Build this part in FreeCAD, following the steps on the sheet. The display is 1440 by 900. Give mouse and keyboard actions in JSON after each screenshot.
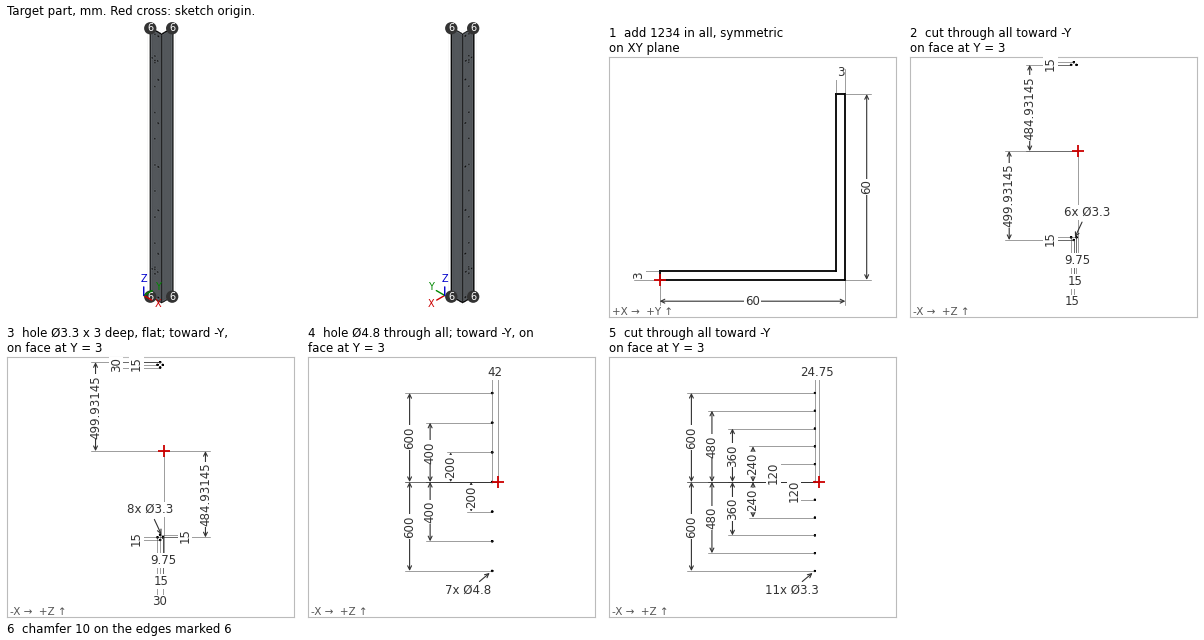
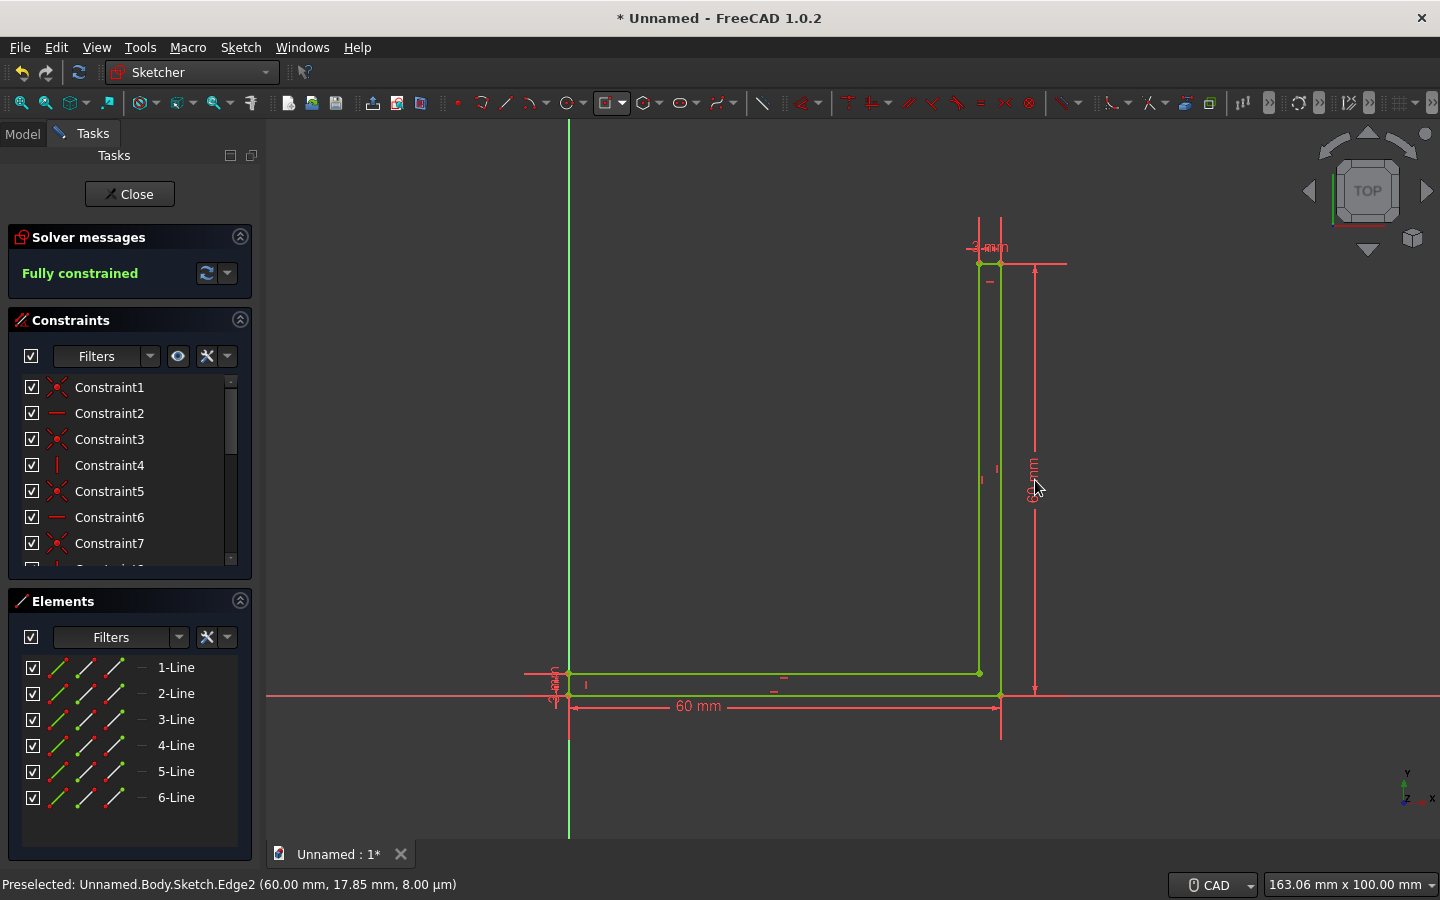
{"action": "left_click", "coordinate": [130, 194]}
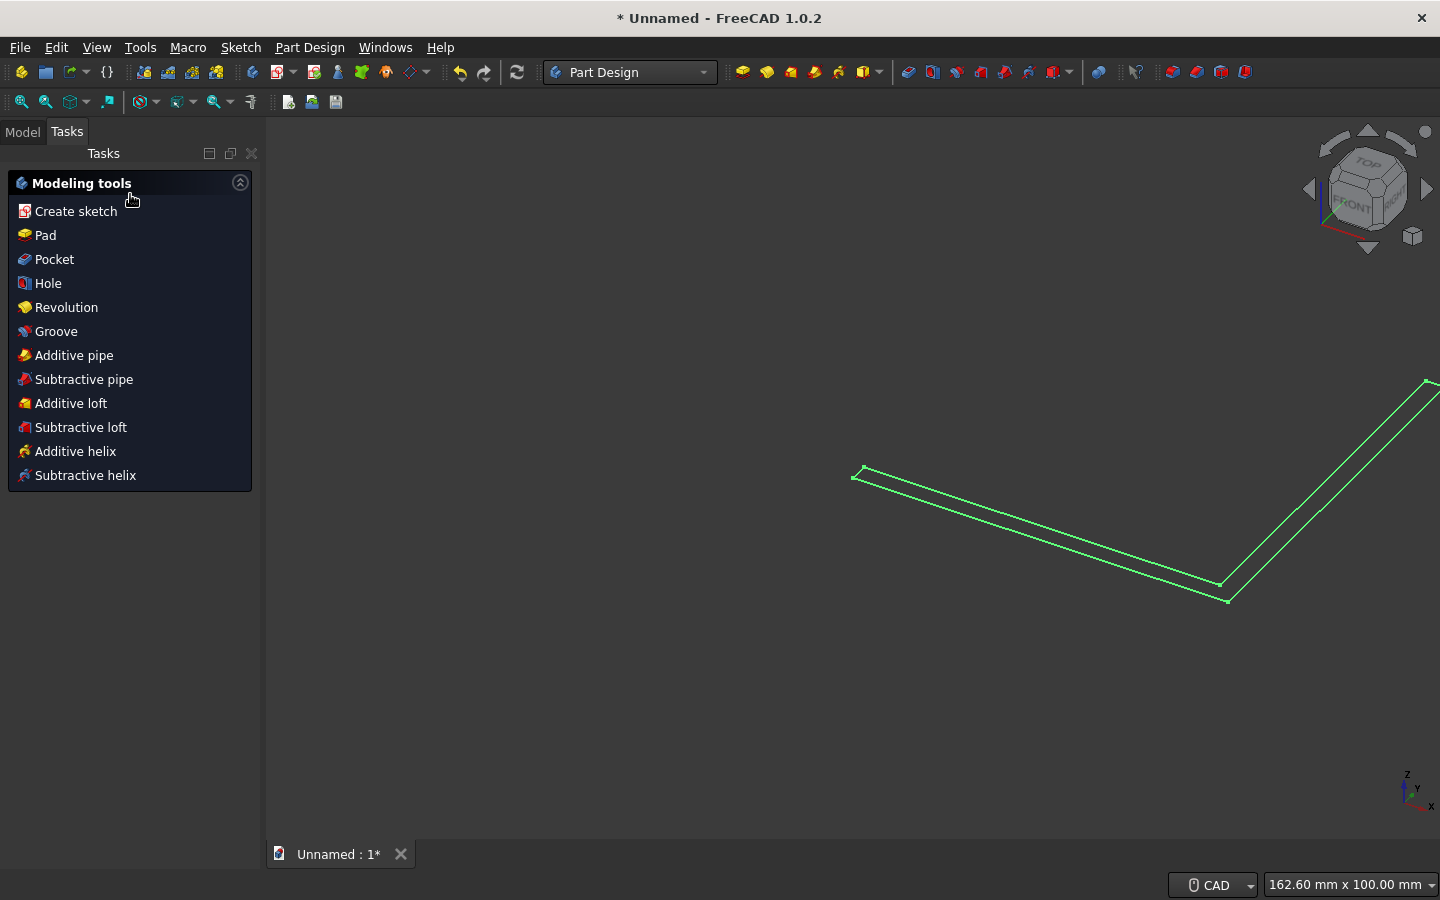
{"action": "left_click", "coordinate": [744, 72]}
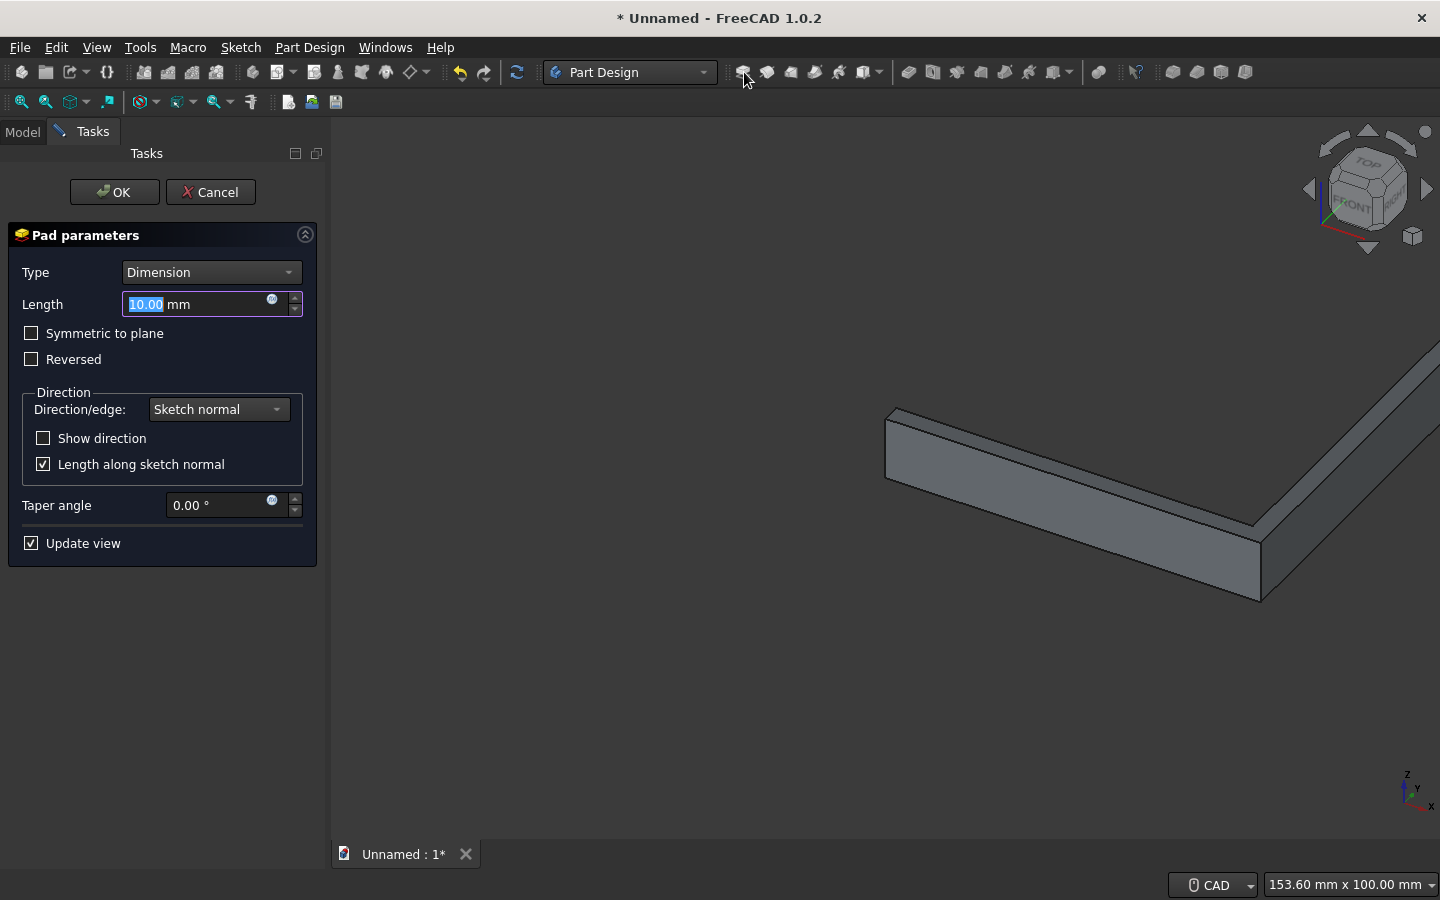
{"action": "type", "text": "1234"}
{"action": "key", "text": "Tab"}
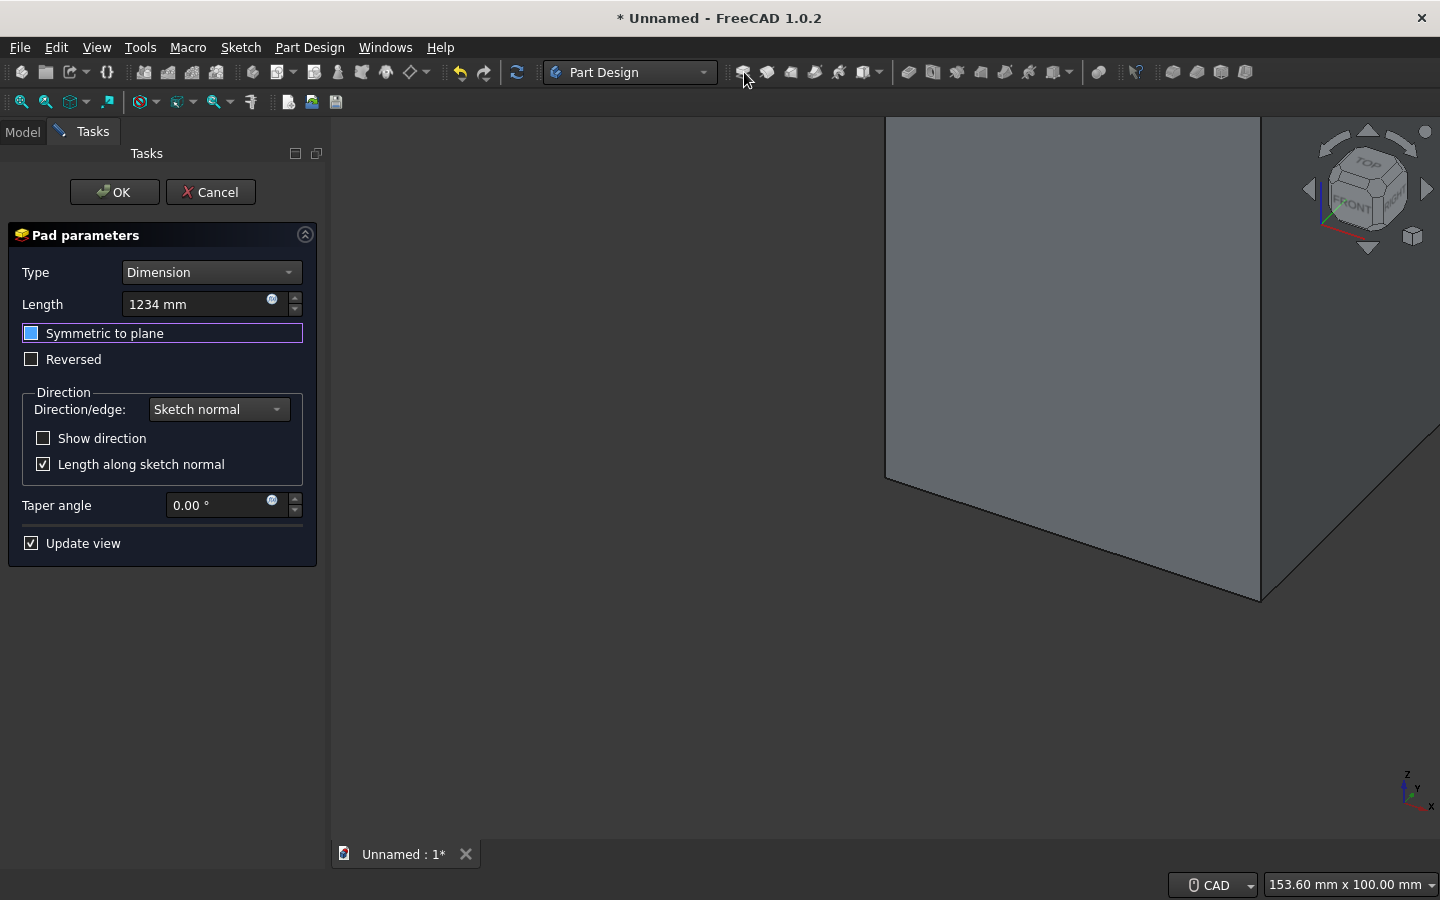
{"action": "left_click", "coordinate": [30, 333]}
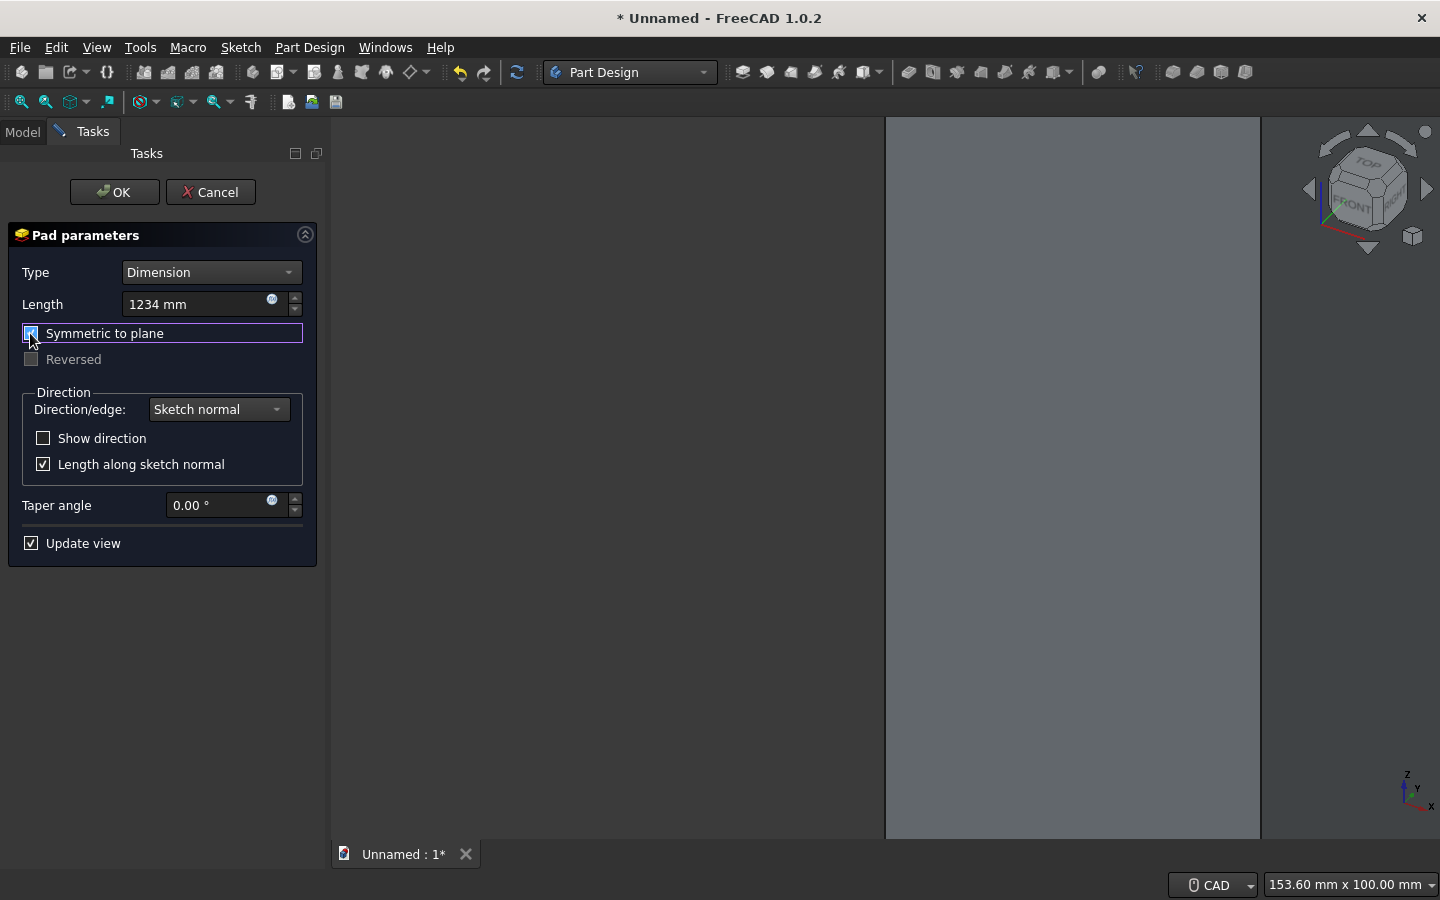
{"action": "left_click", "coordinate": [115, 192]}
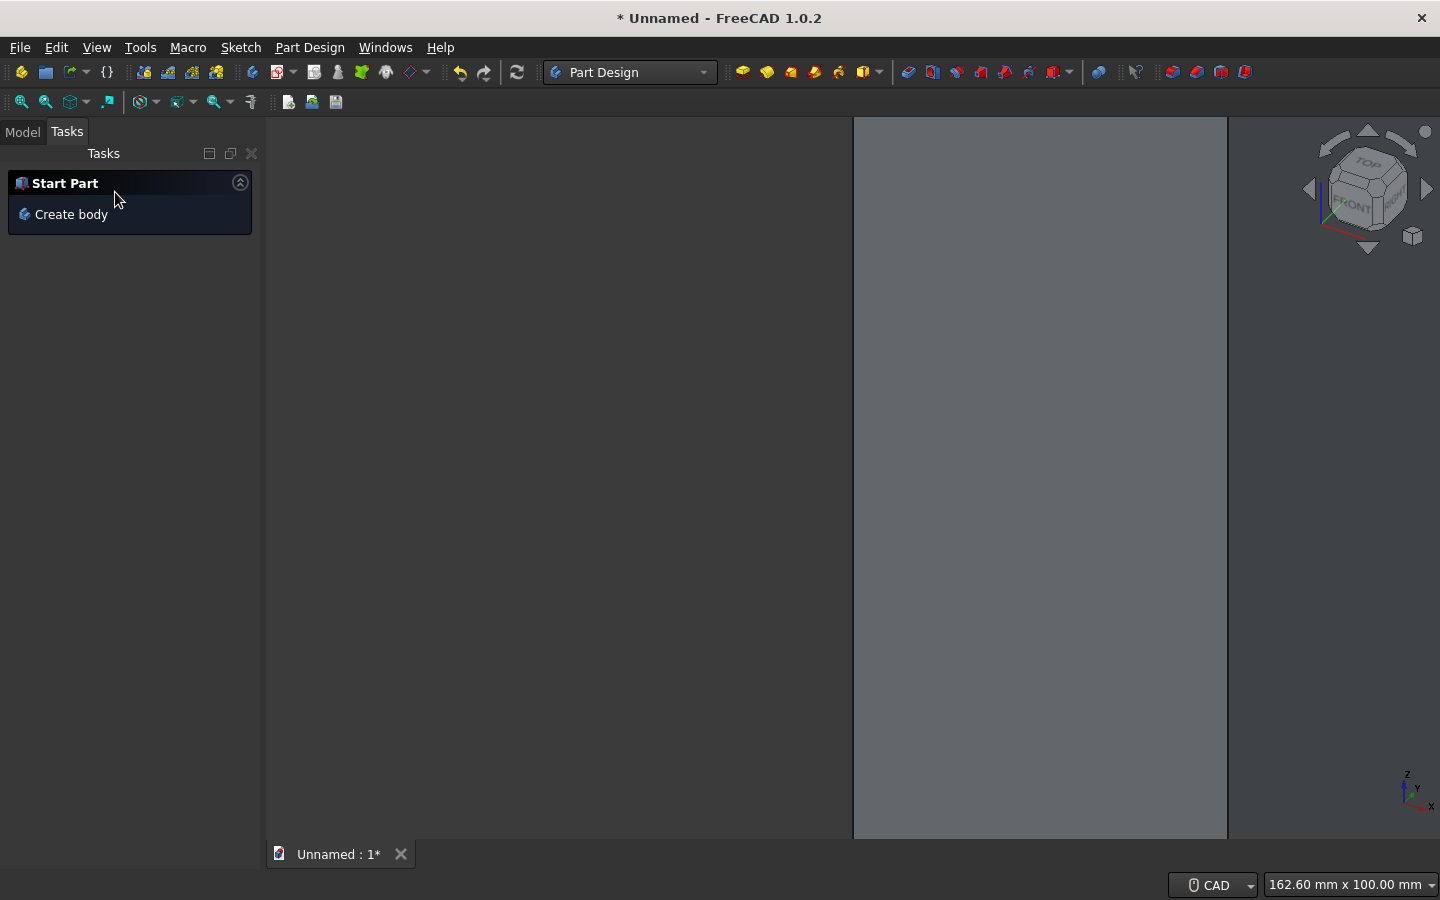
{"action": "left_click", "coordinate": [22, 102]}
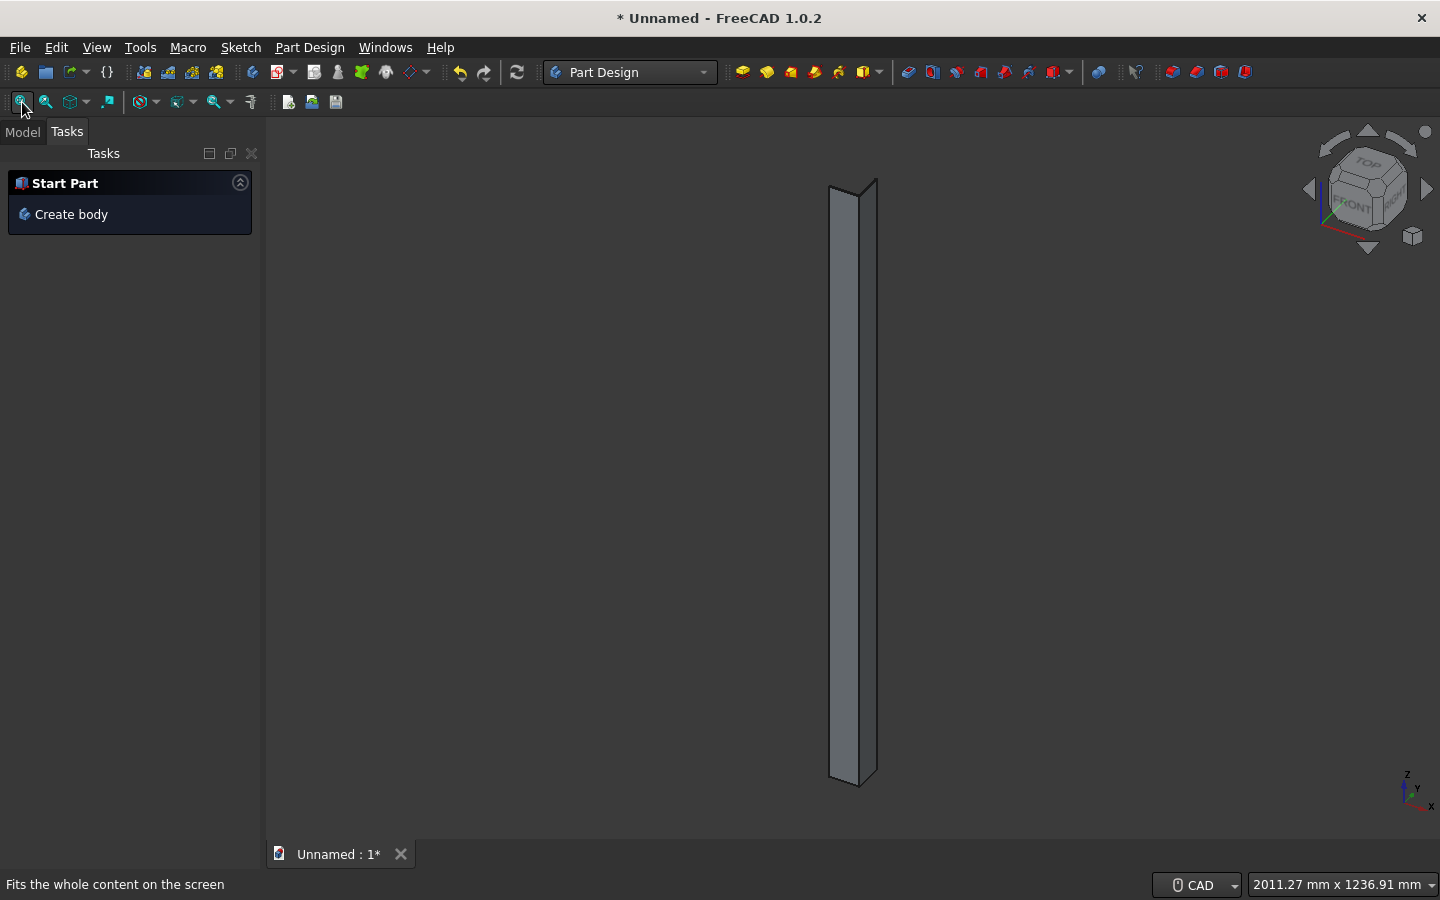
{"action": "key", "text": "4"}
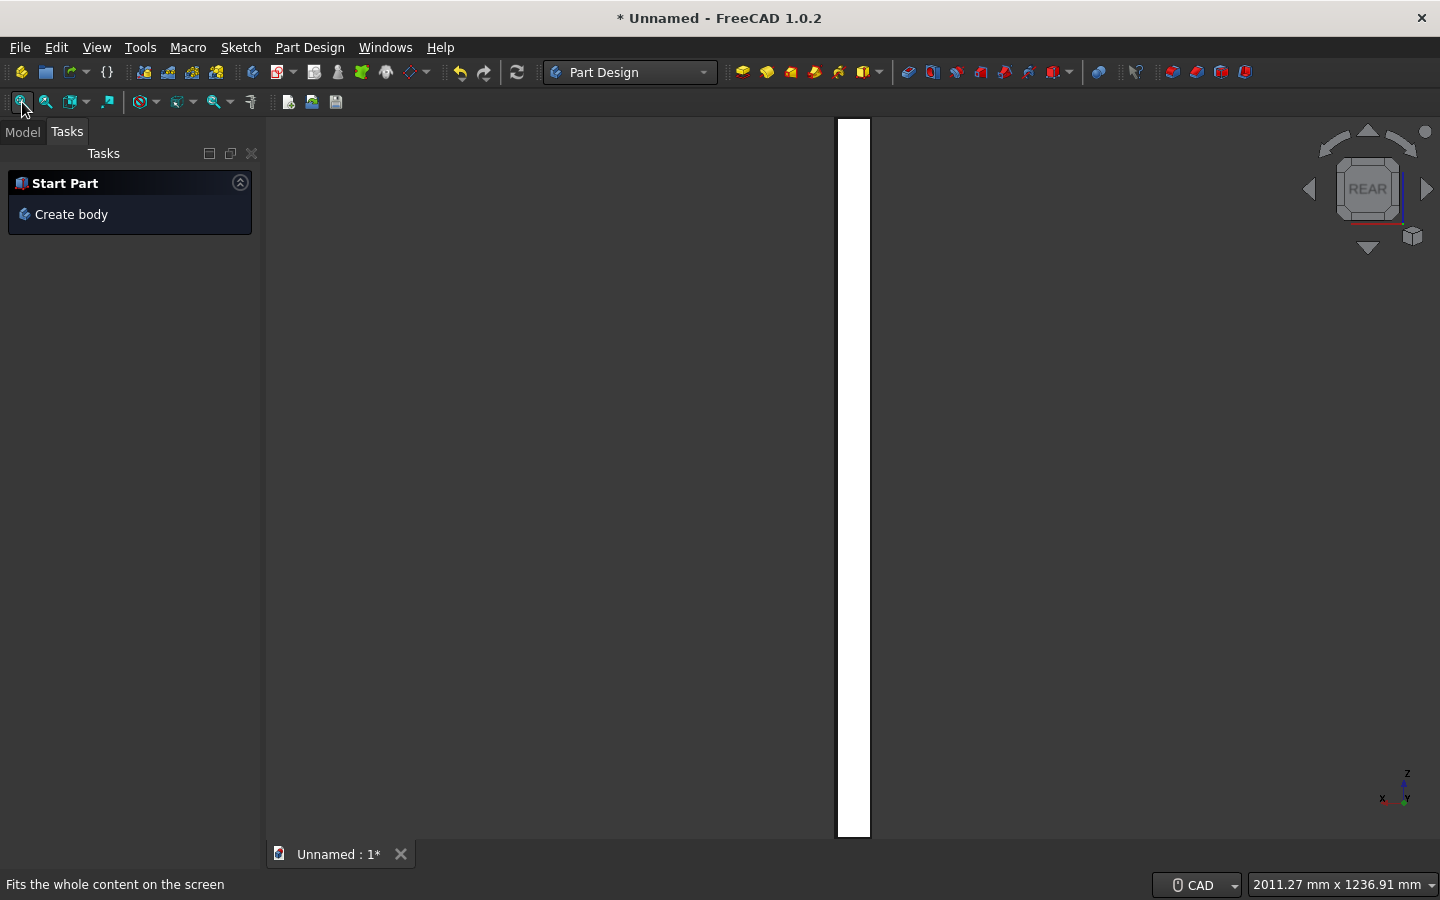
{"action": "left_click", "coordinate": [854, 168]}